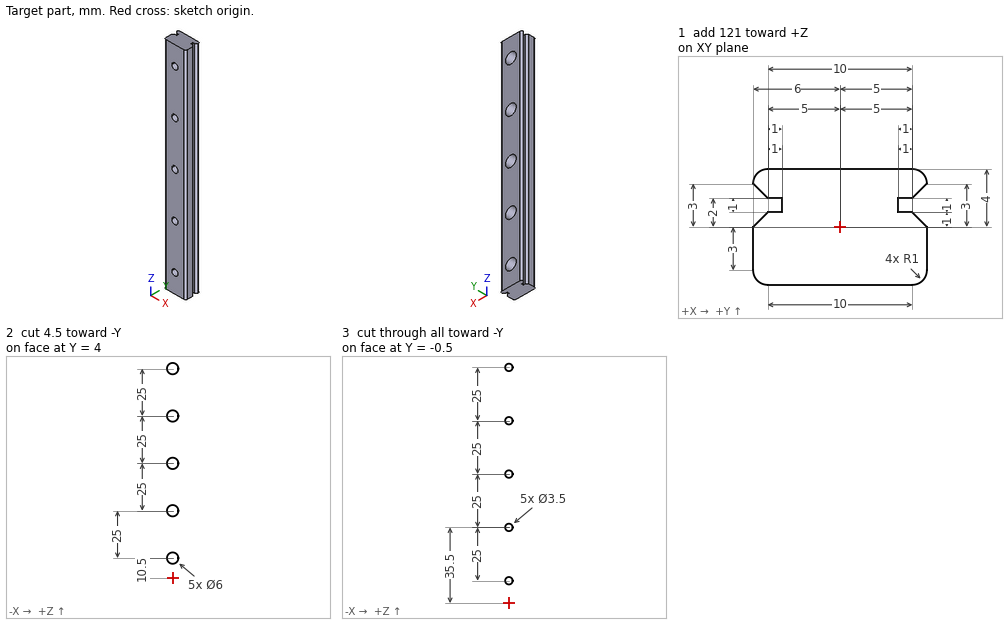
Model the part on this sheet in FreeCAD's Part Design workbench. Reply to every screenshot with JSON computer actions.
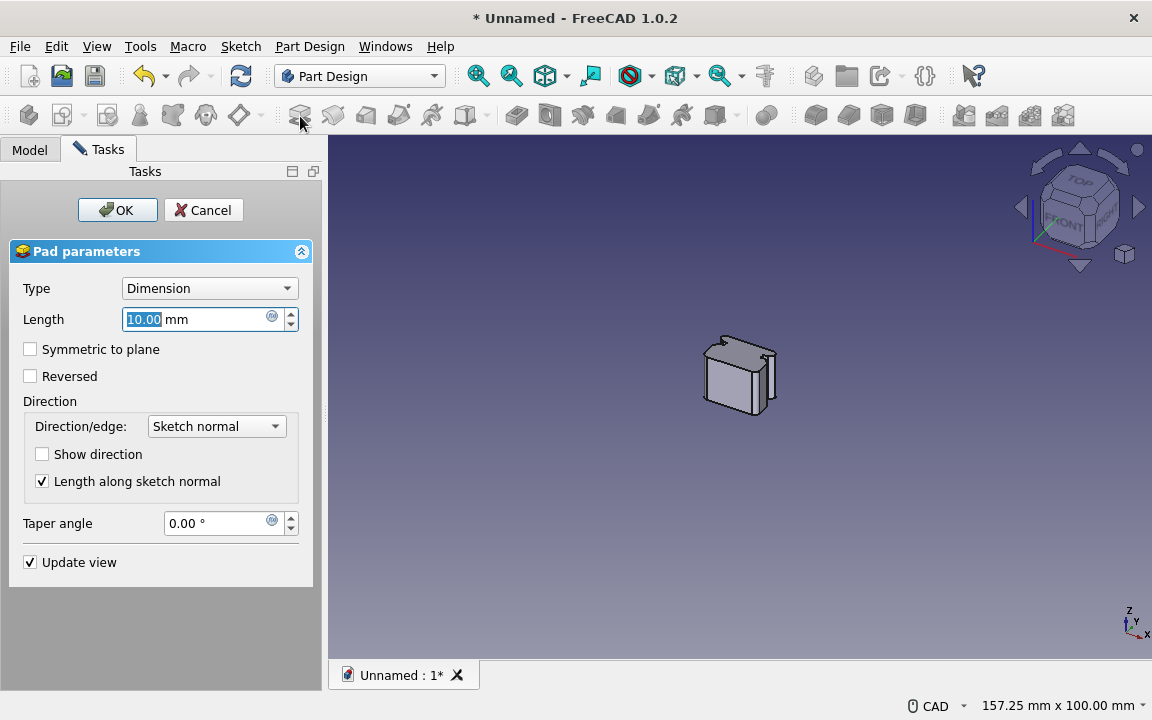
{"action": "type", "text": "121"}
{"action": "key", "text": "Tab"}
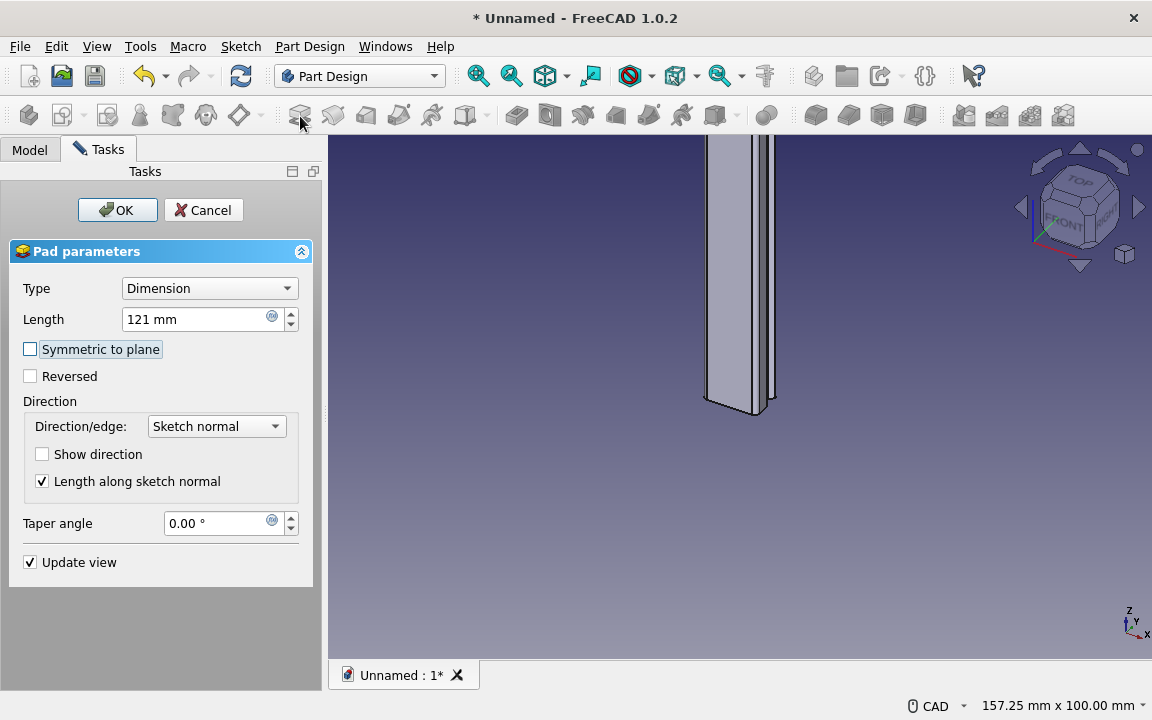
{"action": "left_click", "coordinate": [118, 210]}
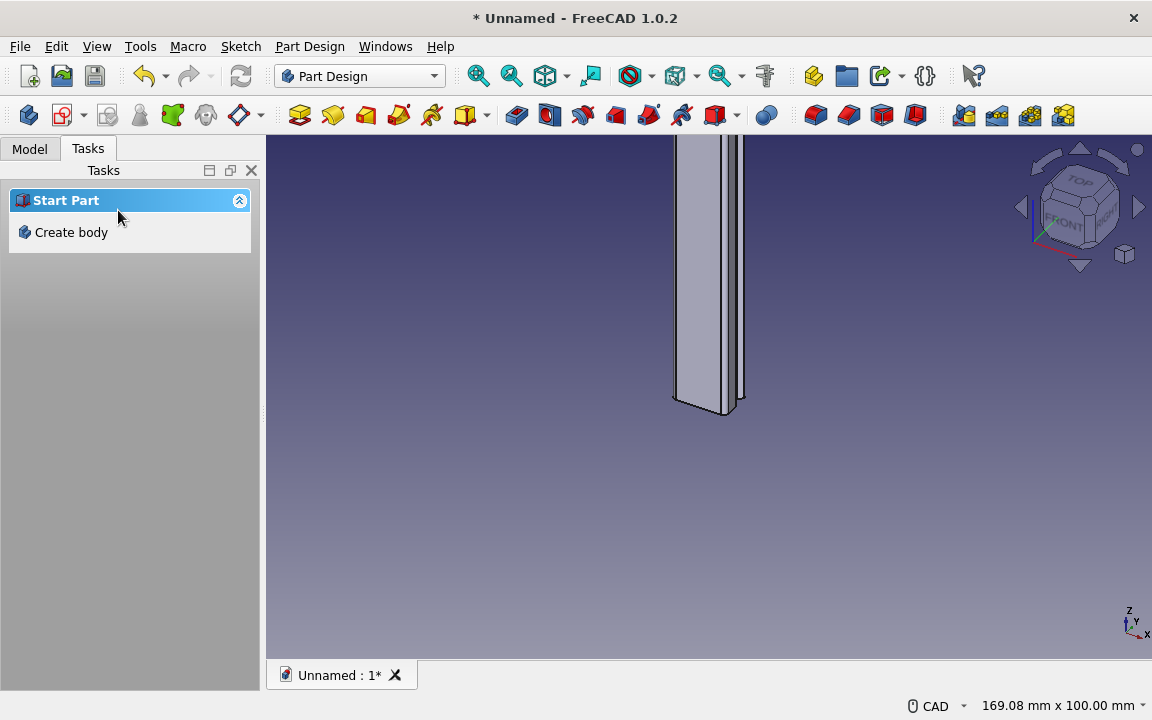
{"action": "left_click", "coordinate": [479, 76]}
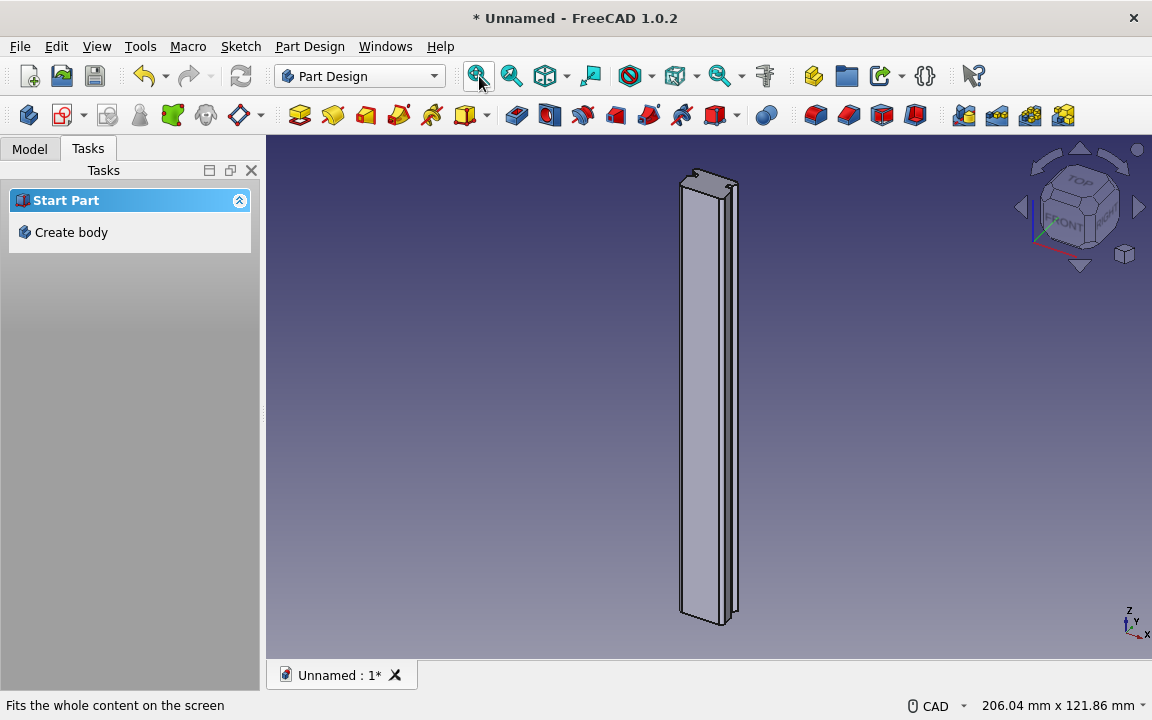
{"action": "key", "text": "4"}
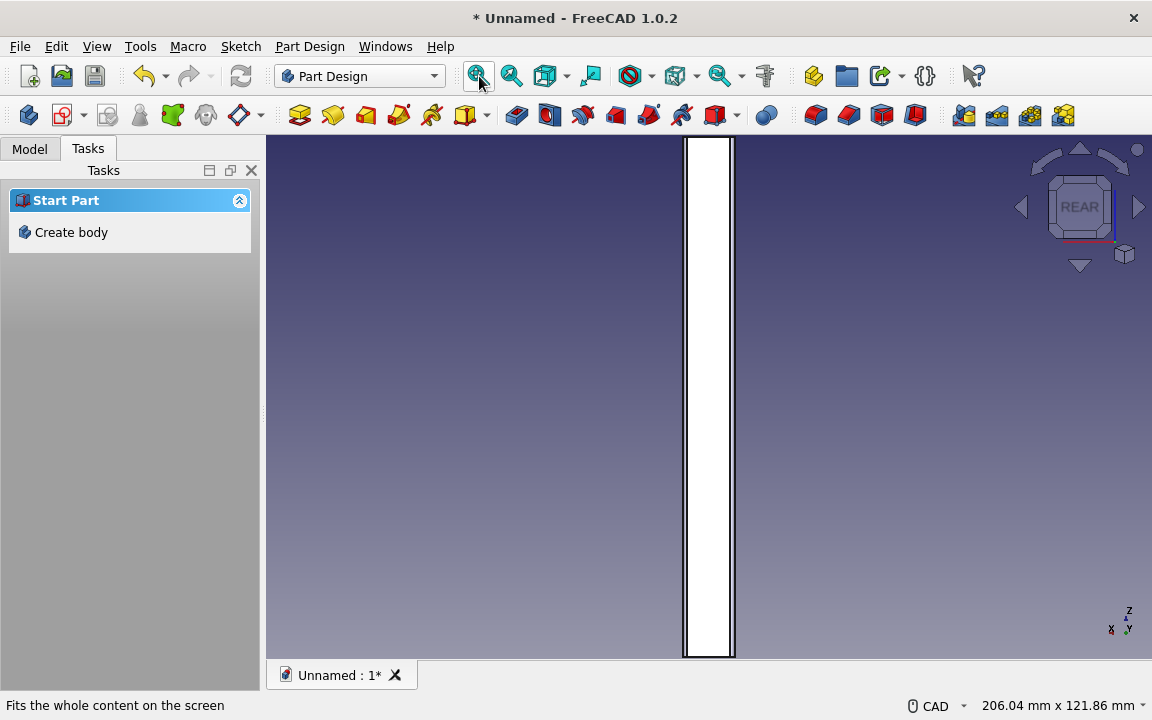
{"action": "left_click", "coordinate": [709, 173]}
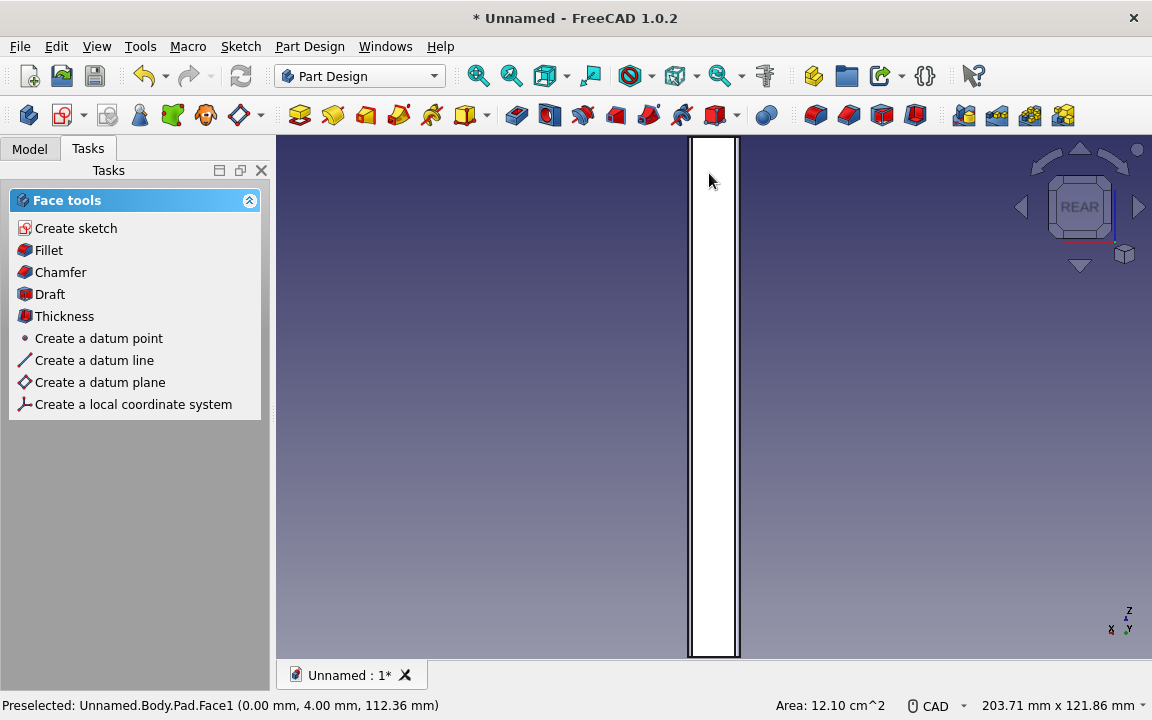
{"action": "left_click", "coordinate": [62, 116]}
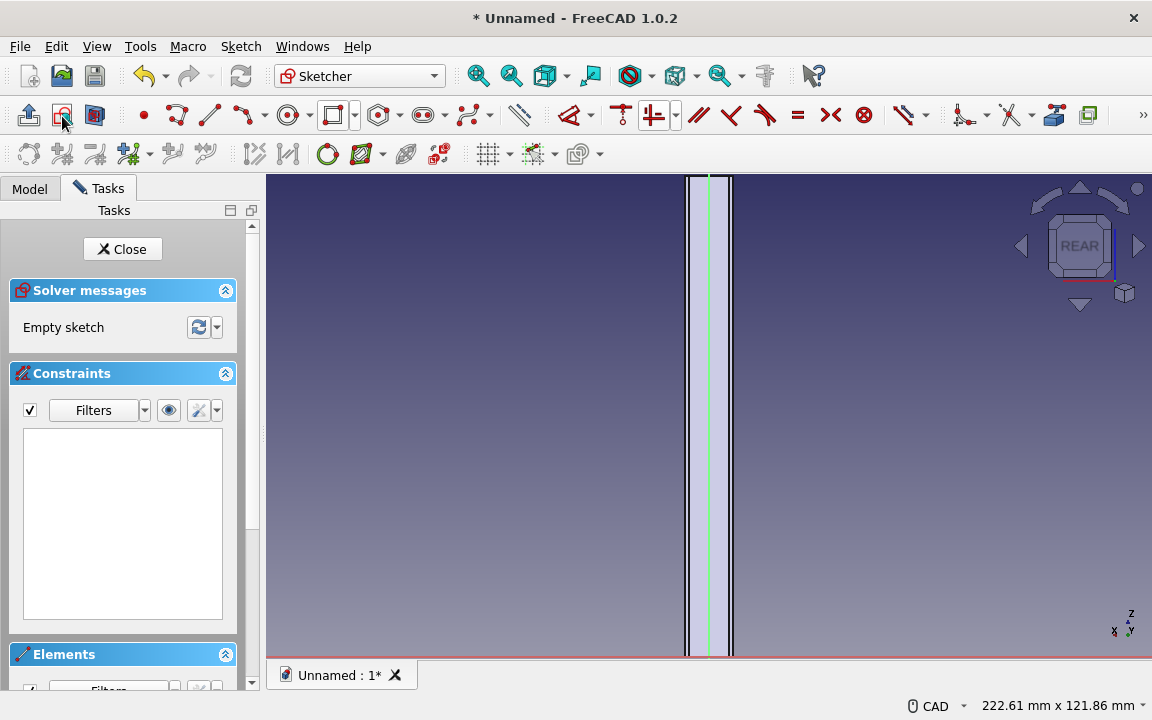
{"action": "scroll", "coordinate": [501, 386], "scroll_direction": "down", "scroll_amount": 2}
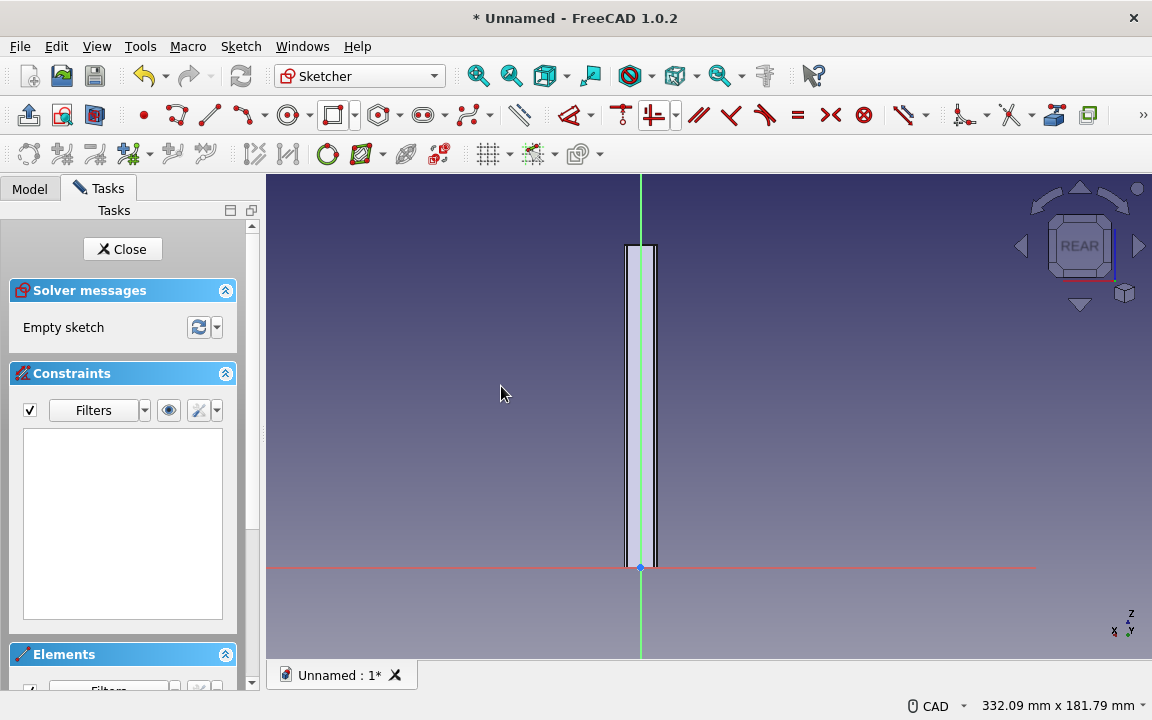
{"action": "left_click", "coordinate": [288, 116]}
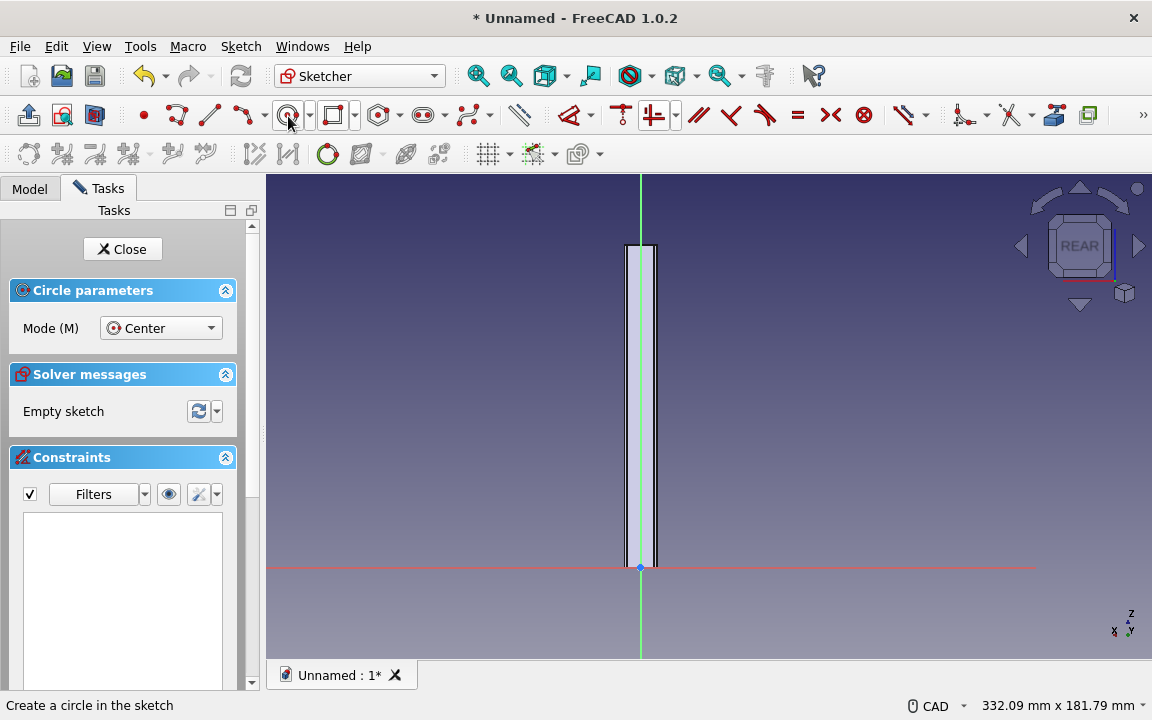
{"action": "scroll", "coordinate": [641, 540], "scroll_direction": "up", "scroll_amount": 6}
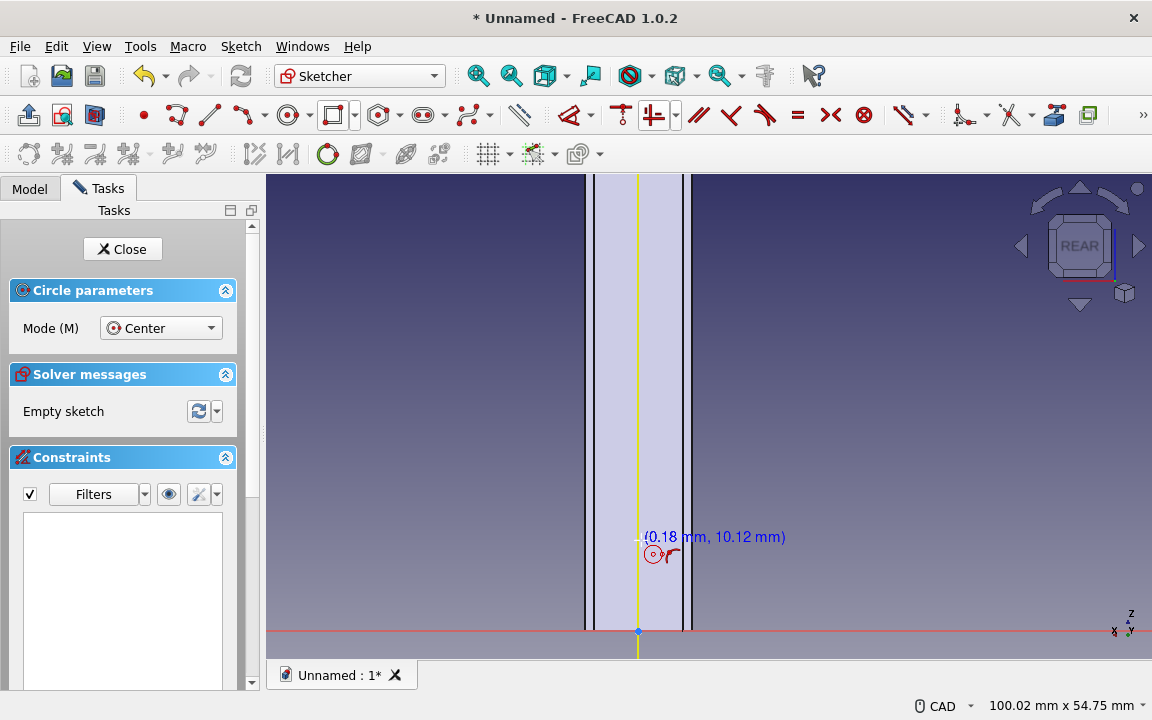
{"action": "left_click", "coordinate": [638, 538]}
{"action": "mouse_move", "coordinate": [657, 519]}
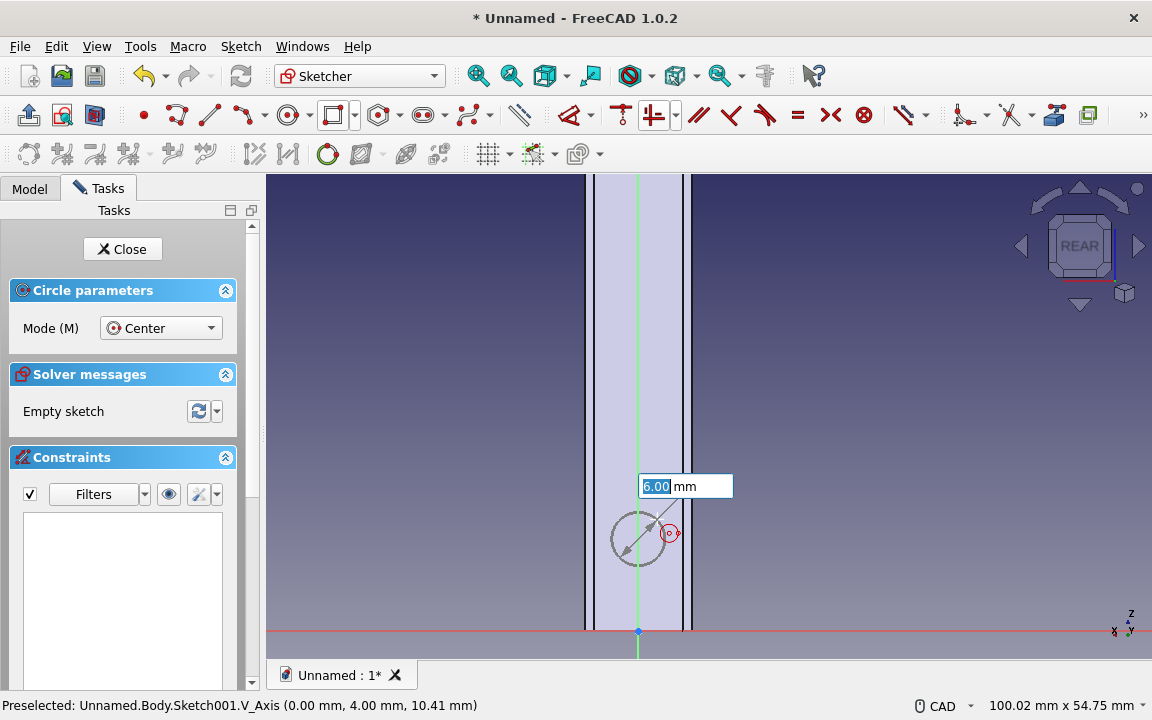
{"action": "type", "text": "6"}
{"action": "key", "text": "Return"}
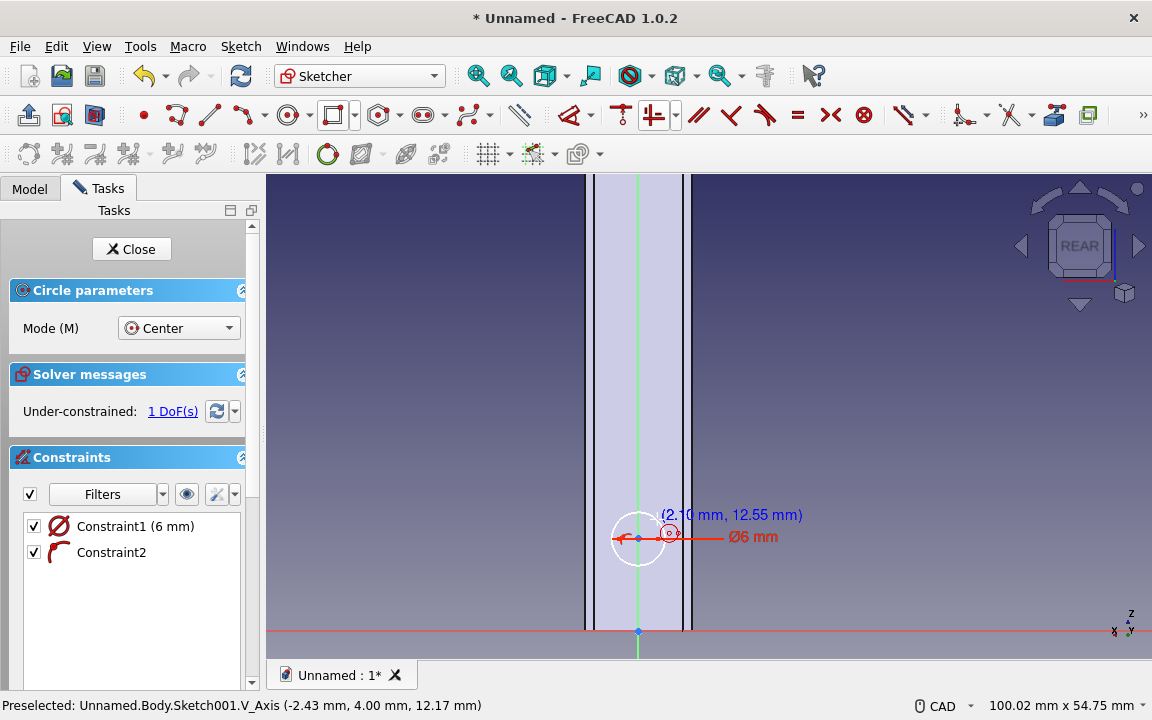
{"action": "left_click", "coordinate": [638, 317]}
{"action": "mouse_move", "coordinate": [657, 298]}